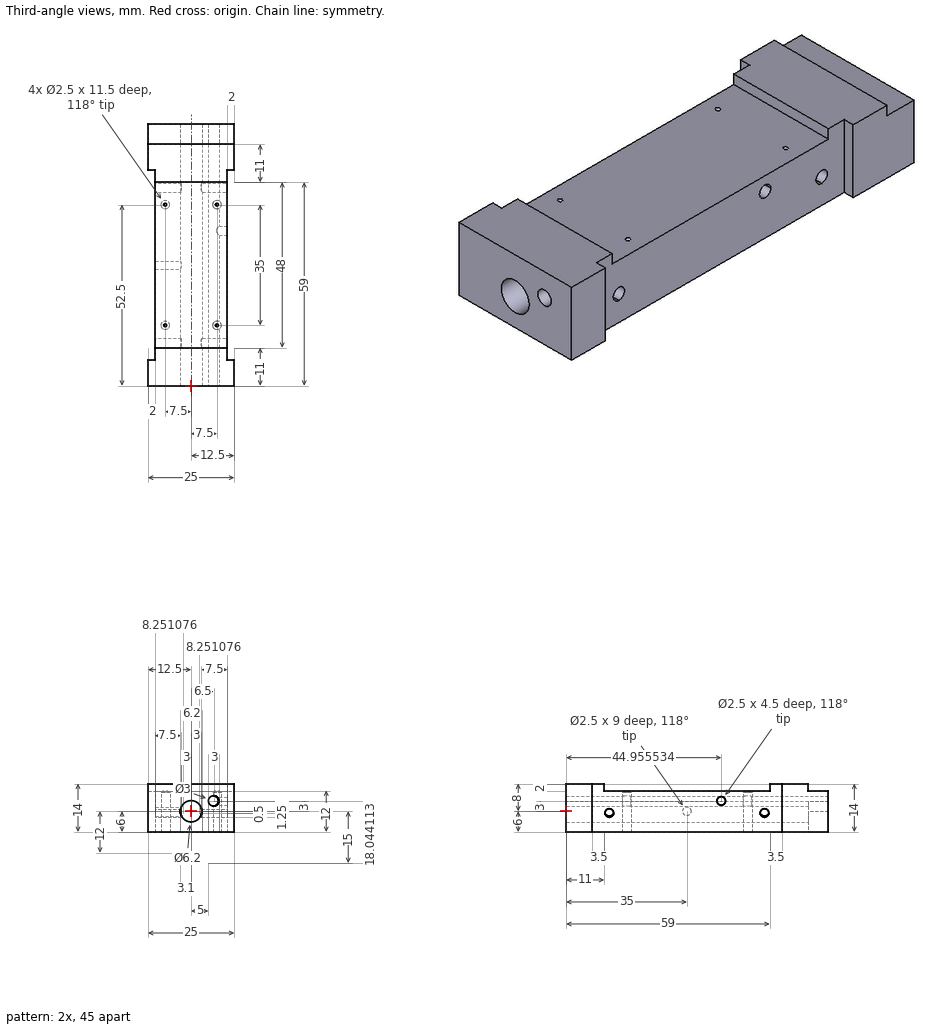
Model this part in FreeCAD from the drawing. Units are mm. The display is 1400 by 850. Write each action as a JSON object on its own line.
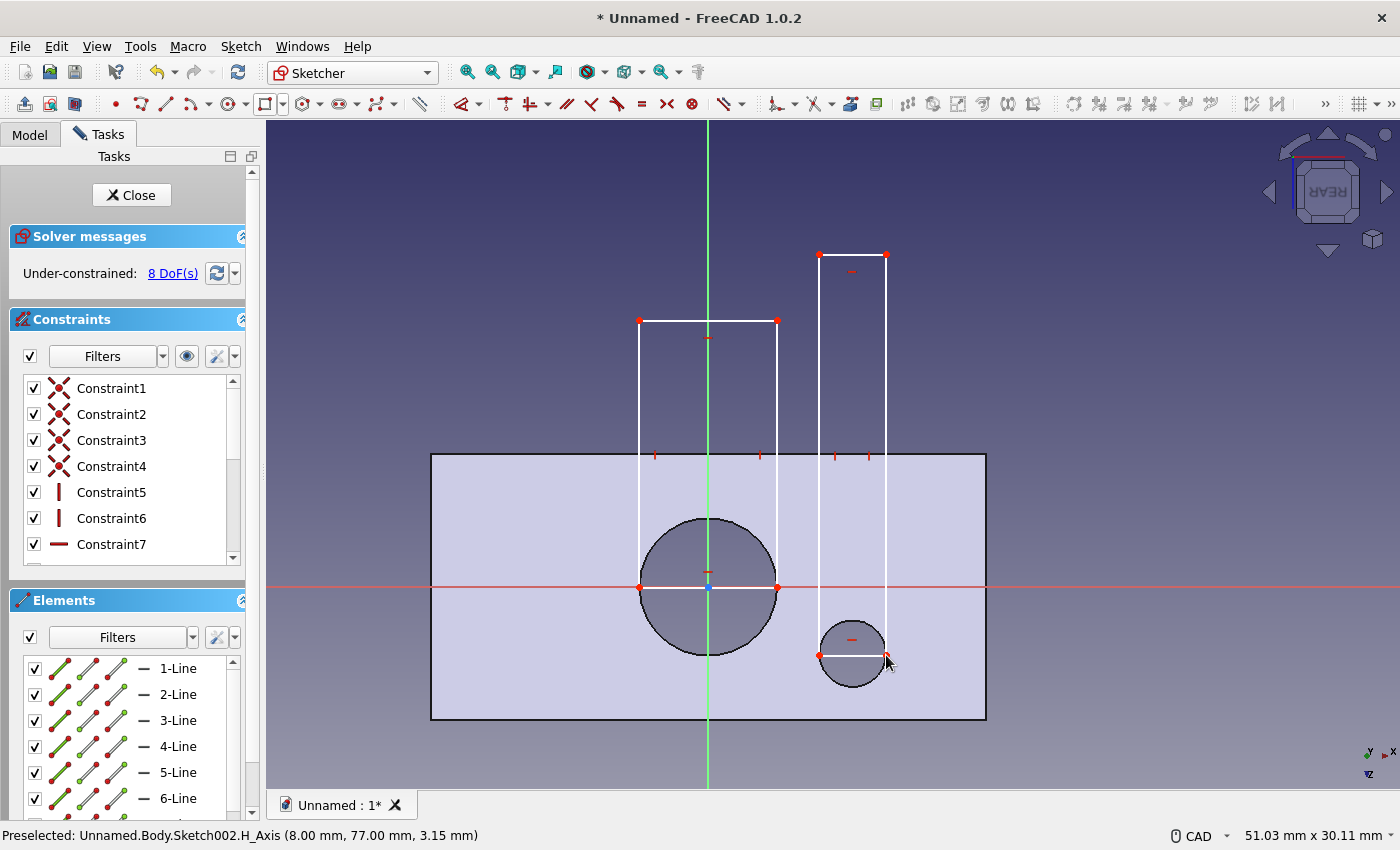
{"action": "left_click", "coordinate": [639, 588]}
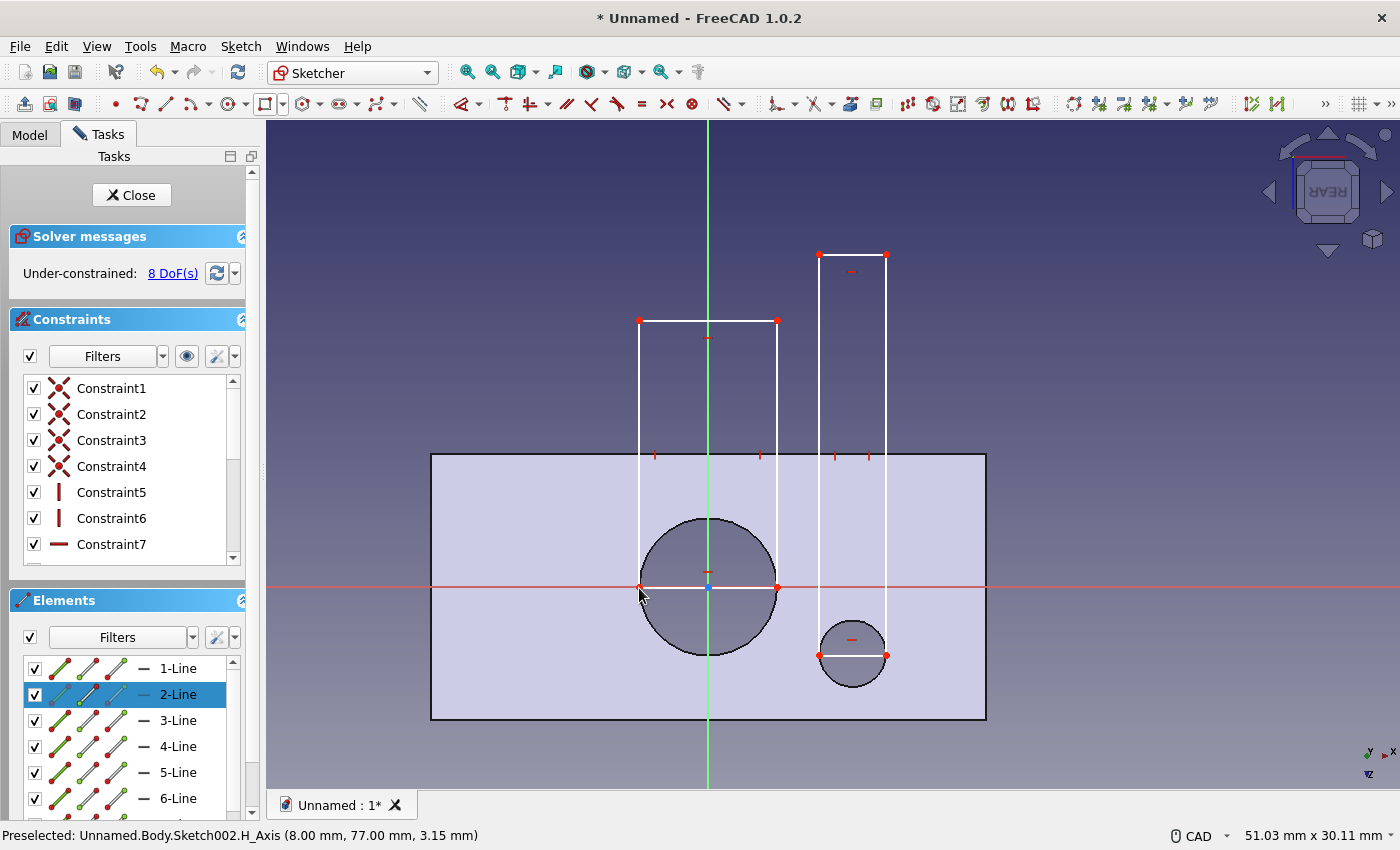
{"action": "left_click", "coordinate": [361, 587]}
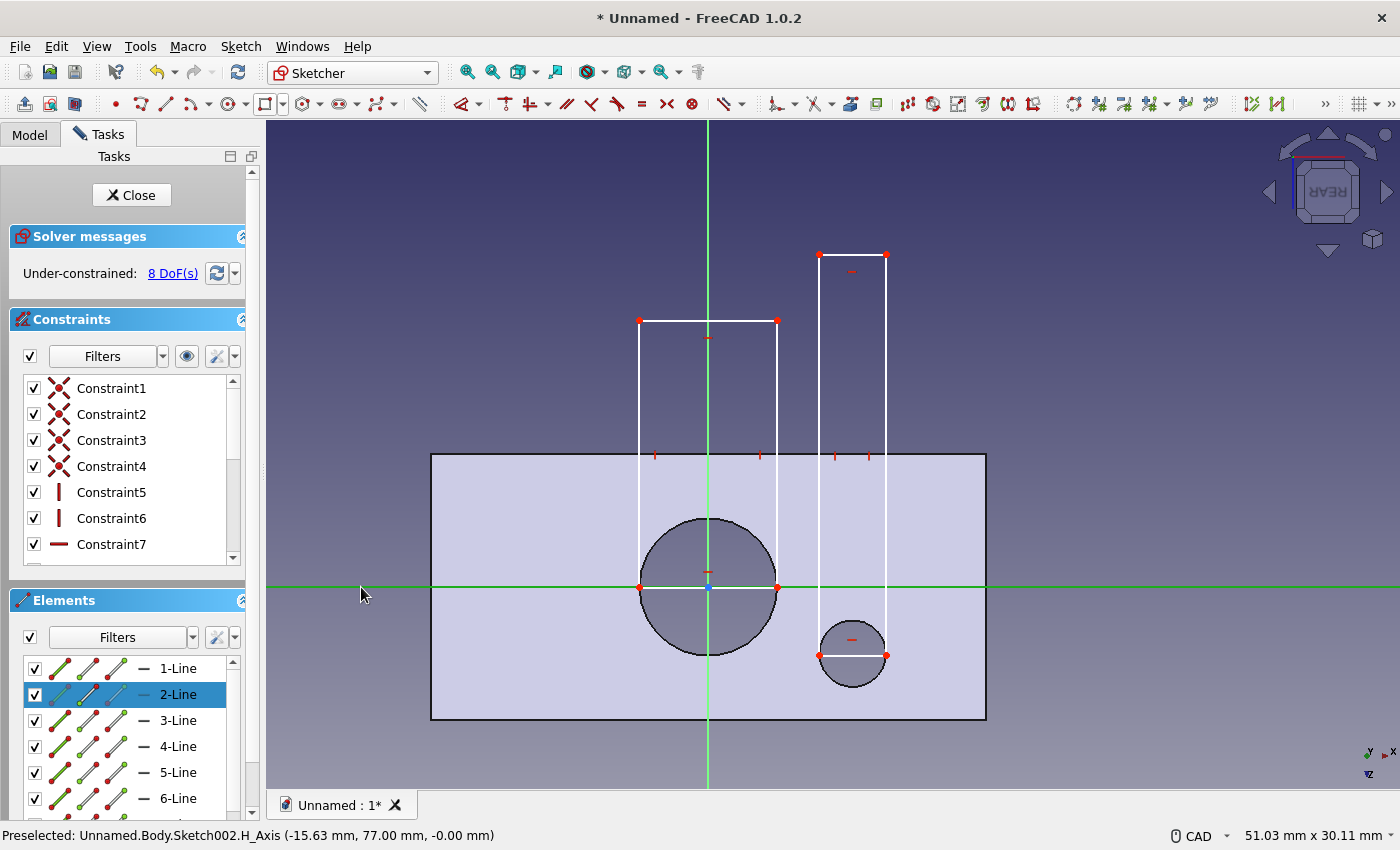
{"action": "left_click", "coordinate": [505, 104]}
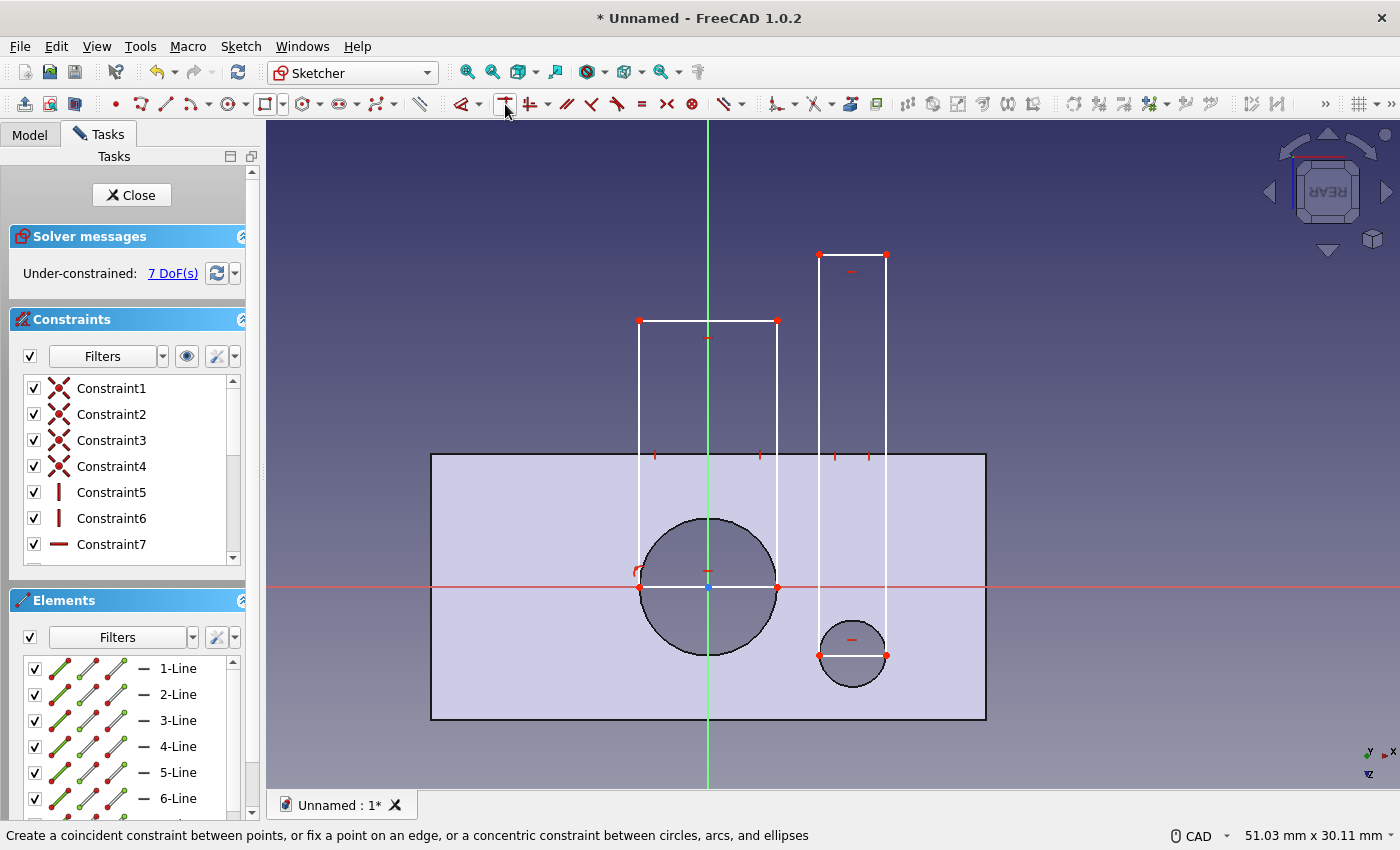
{"action": "left_click", "coordinate": [460, 104]}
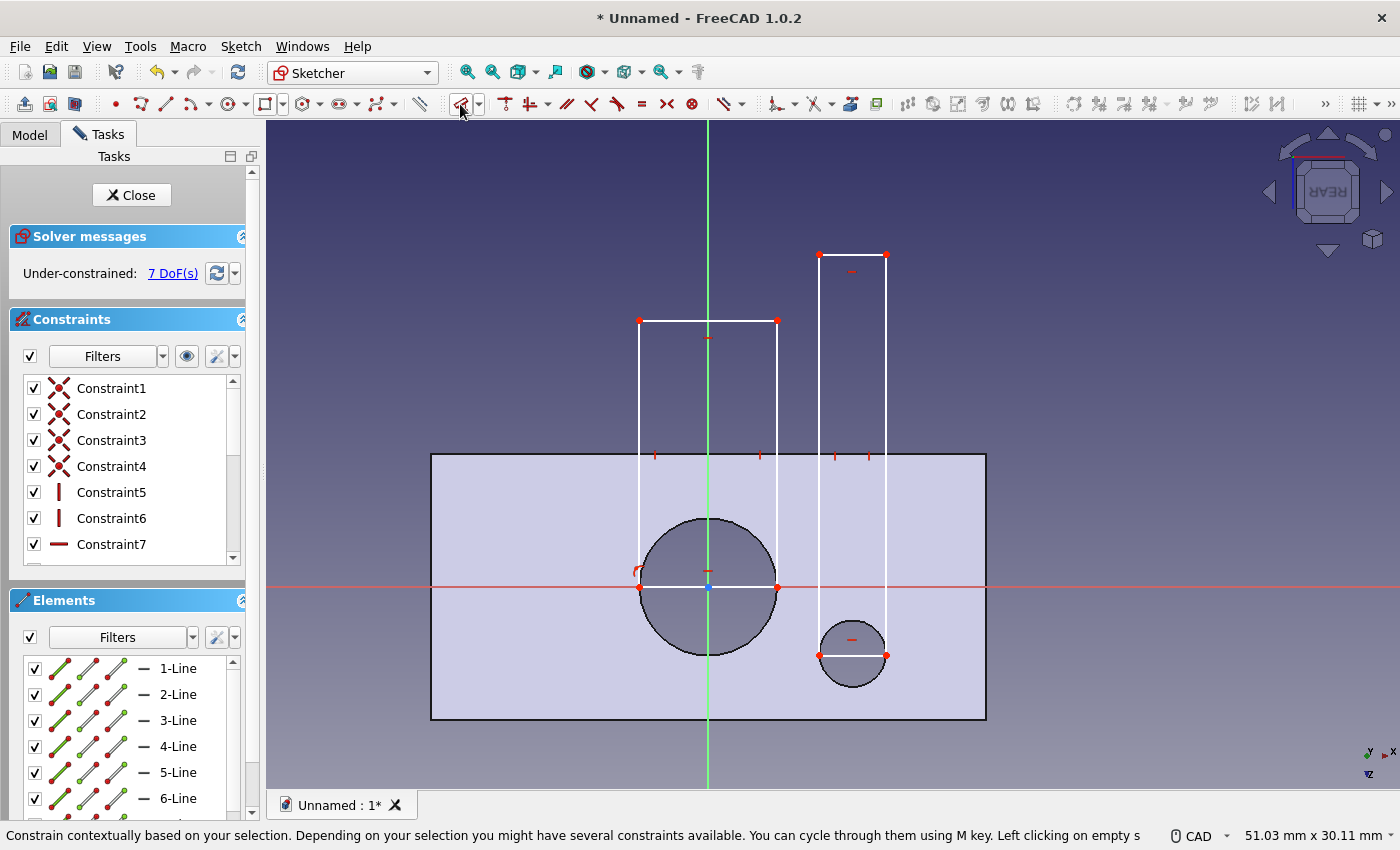
{"action": "left_click", "coordinate": [839, 656]}
{"action": "left_click", "coordinate": [852, 690]}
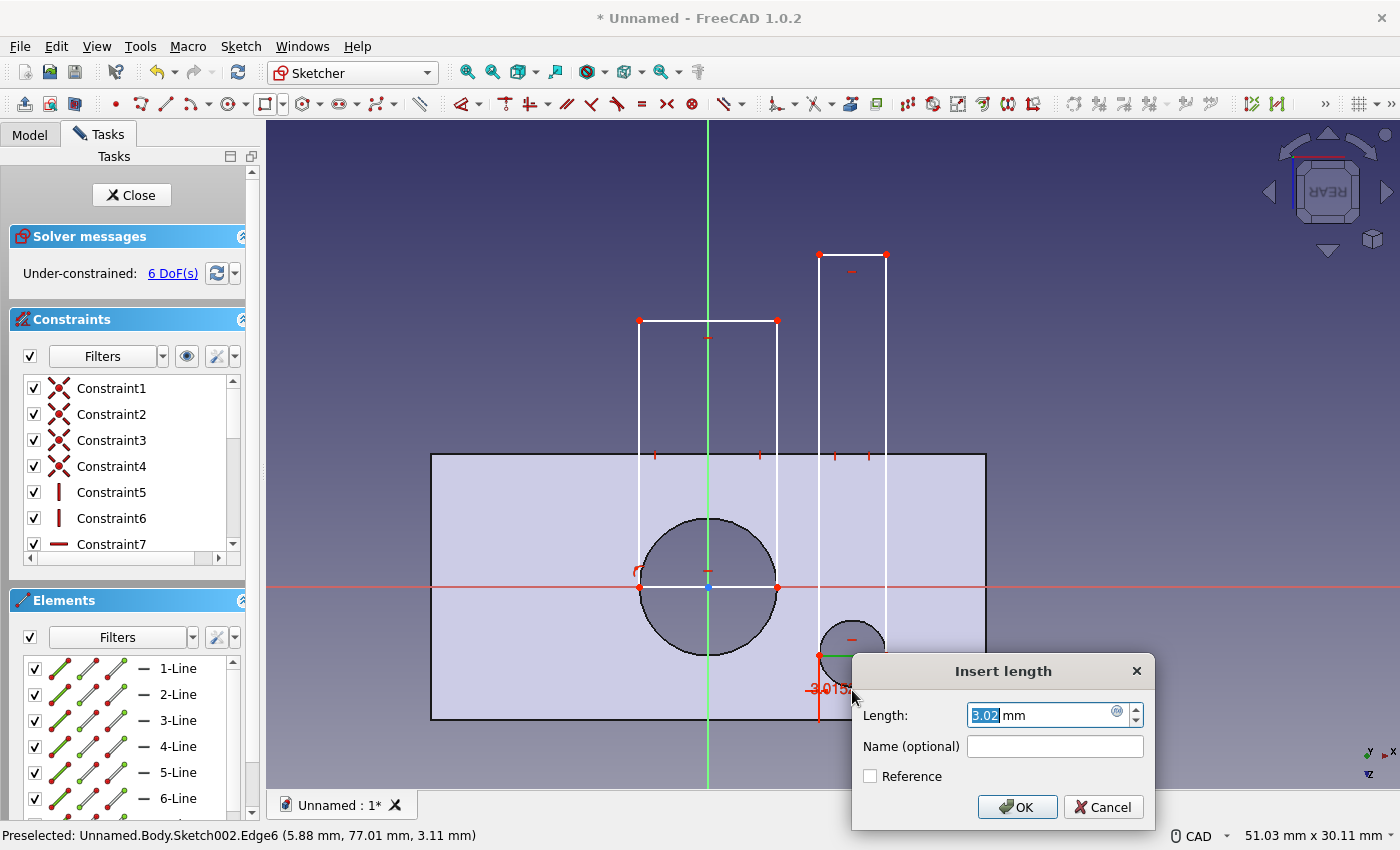
{"action": "type", "text": "3"}
{"action": "key", "text": "Return"}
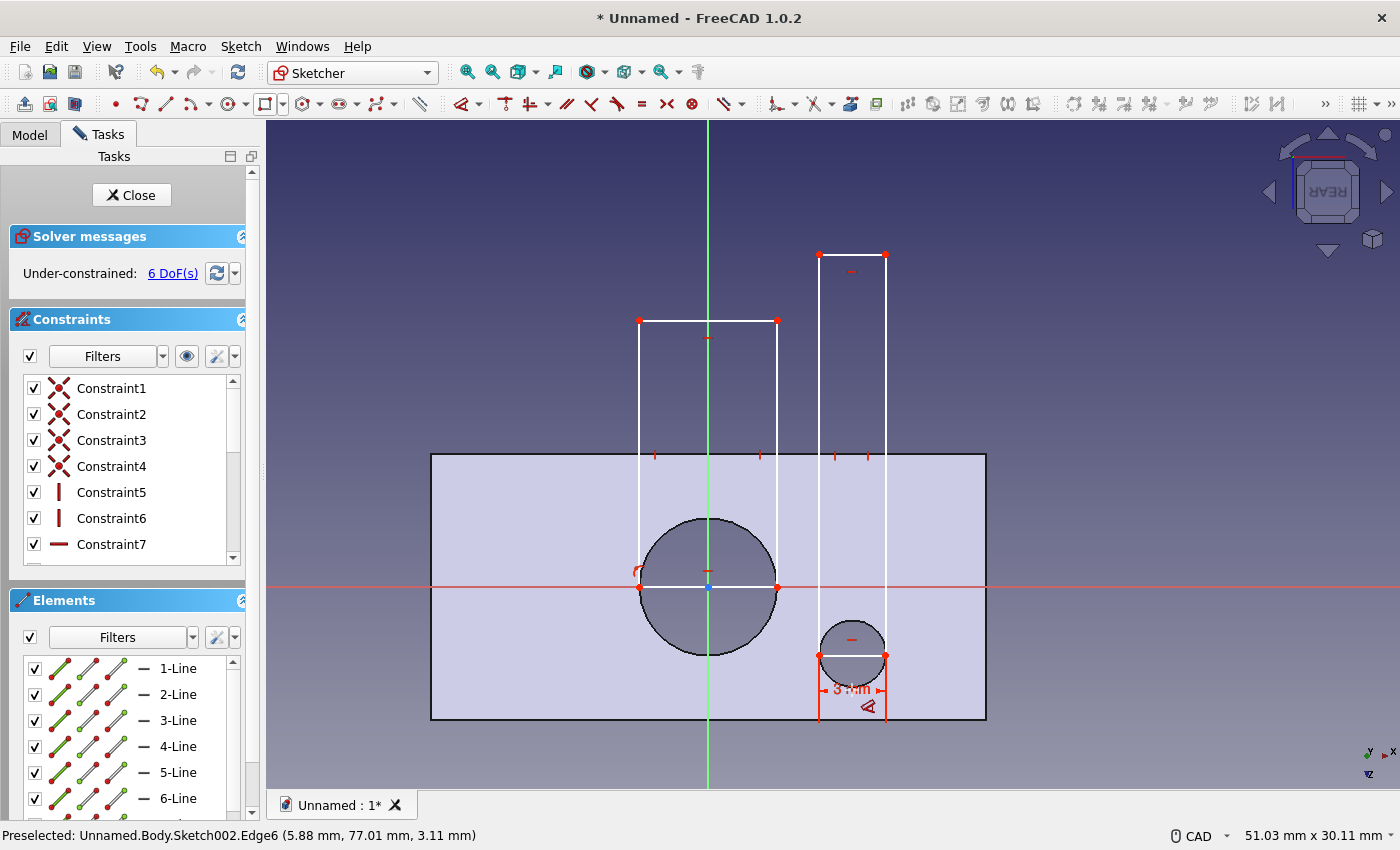
{"action": "left_click", "coordinate": [639, 401]}
{"action": "left_click", "coordinate": [605, 454]}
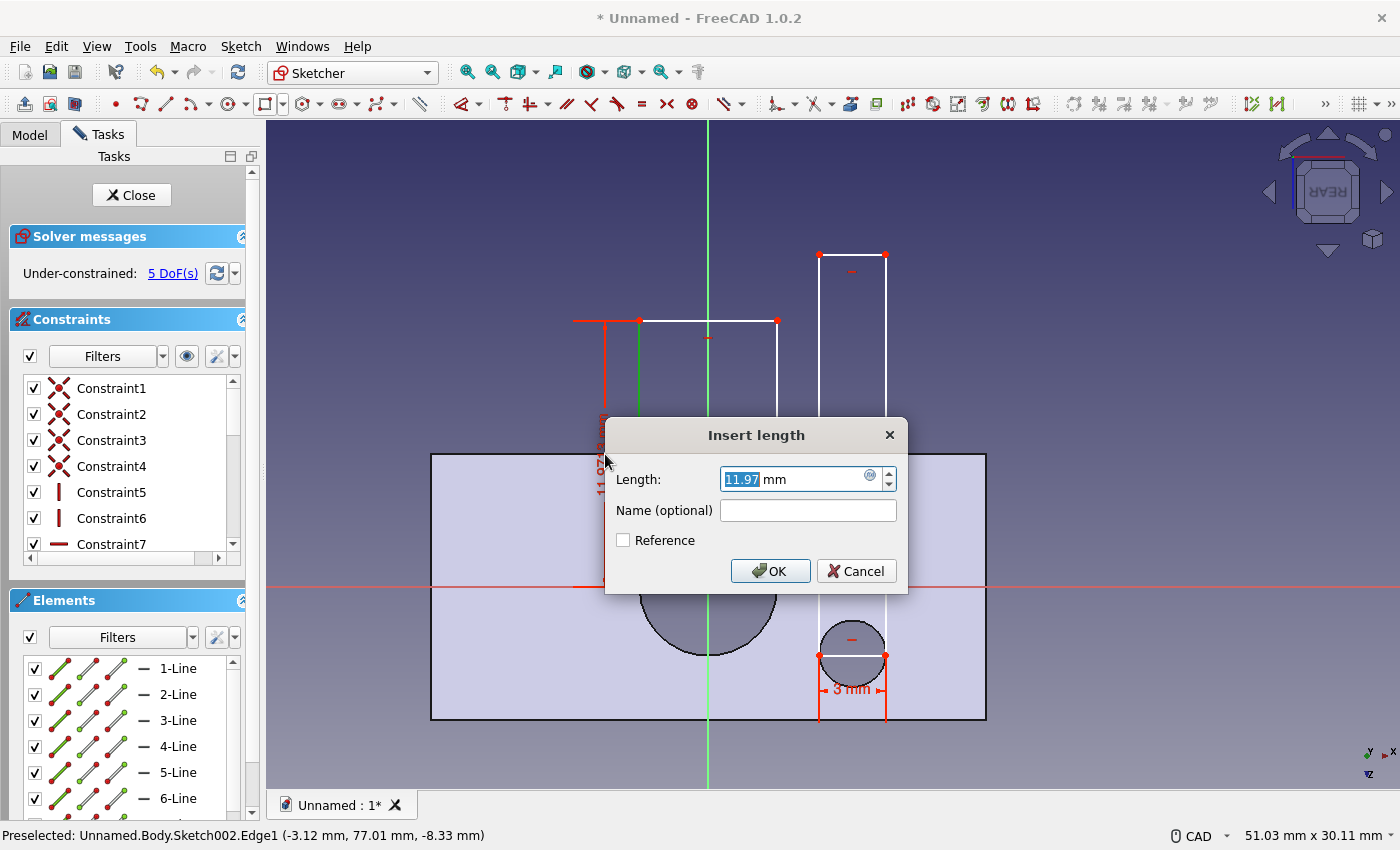
{"action": "type", "text": "12"}
{"action": "key", "text": "Return"}